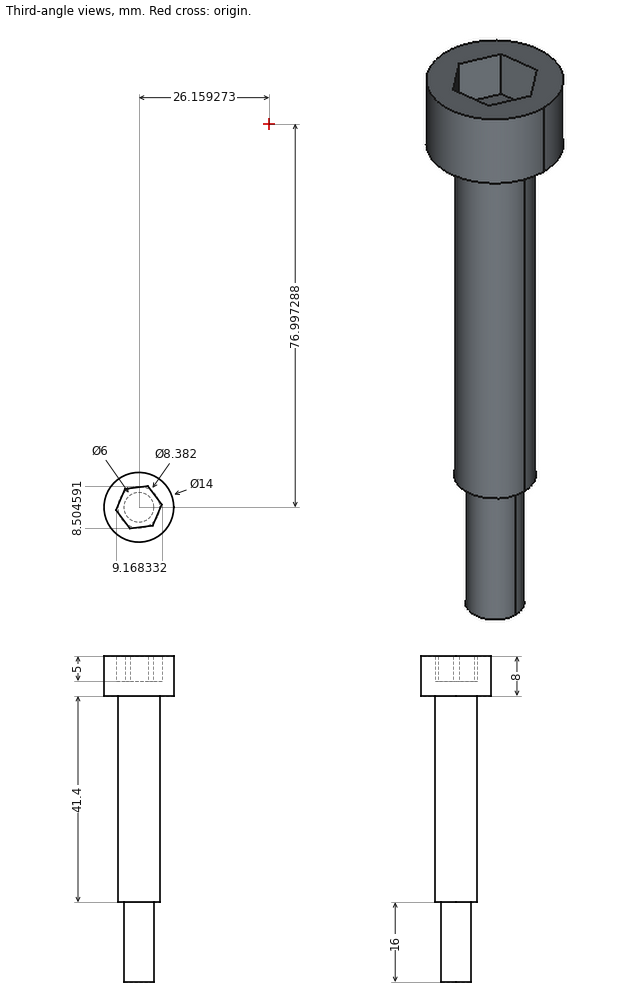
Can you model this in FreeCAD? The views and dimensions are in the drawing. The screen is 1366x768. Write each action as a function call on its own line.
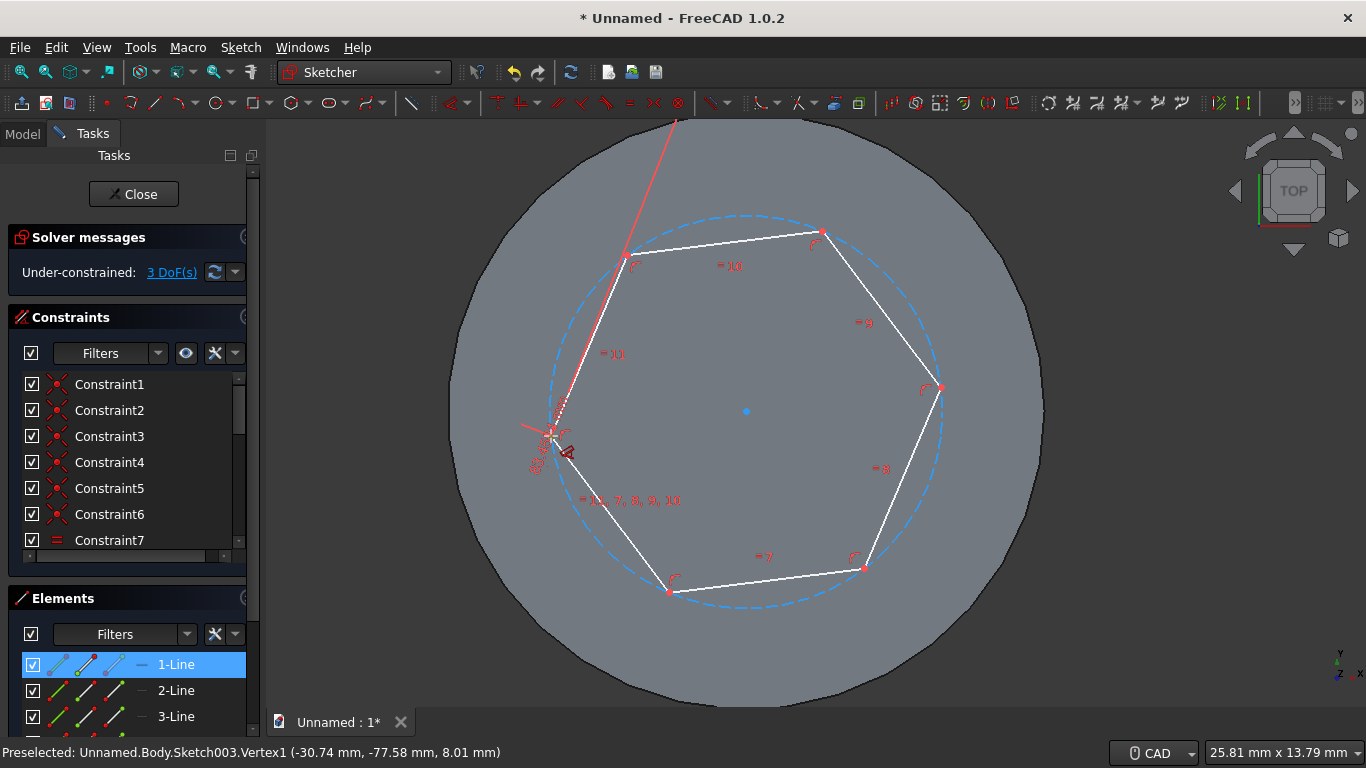
click(941, 388)
click(746, 470)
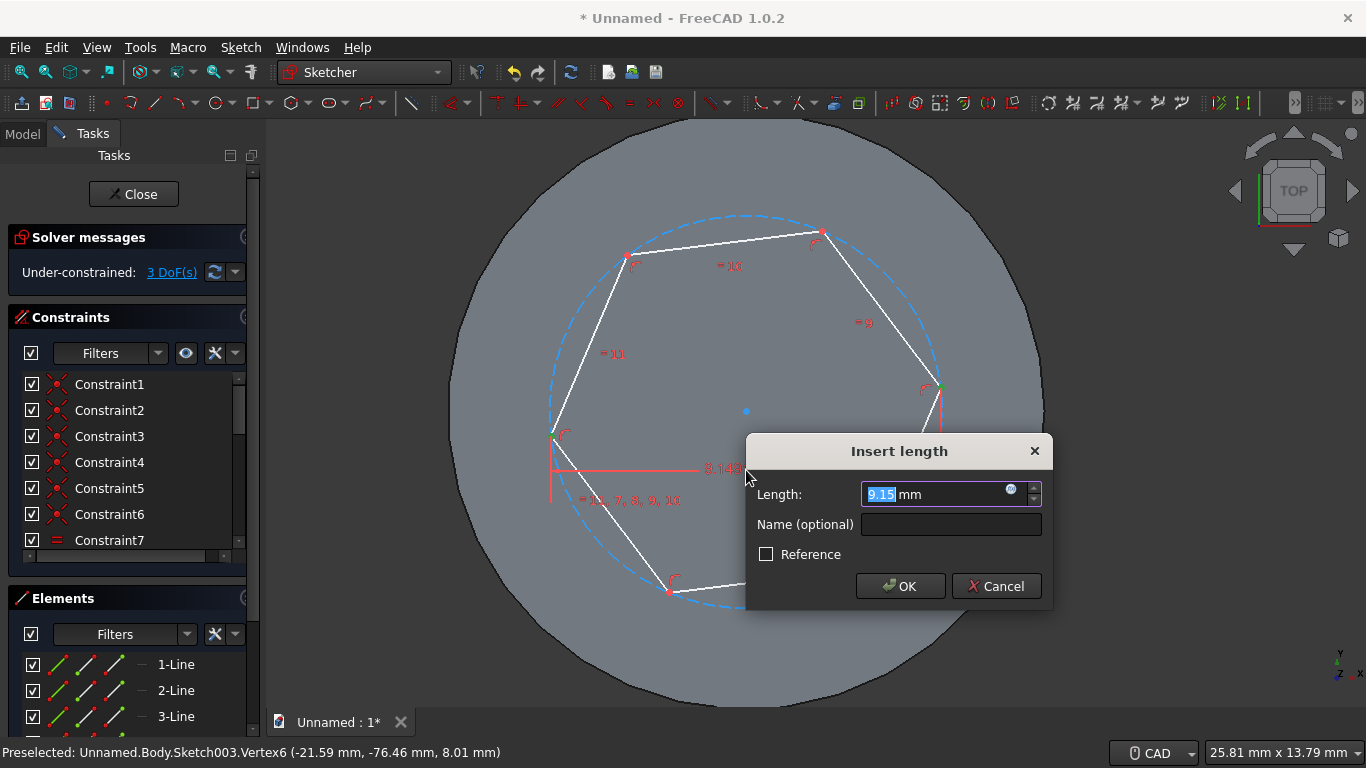
text(9.168332)
key(Return)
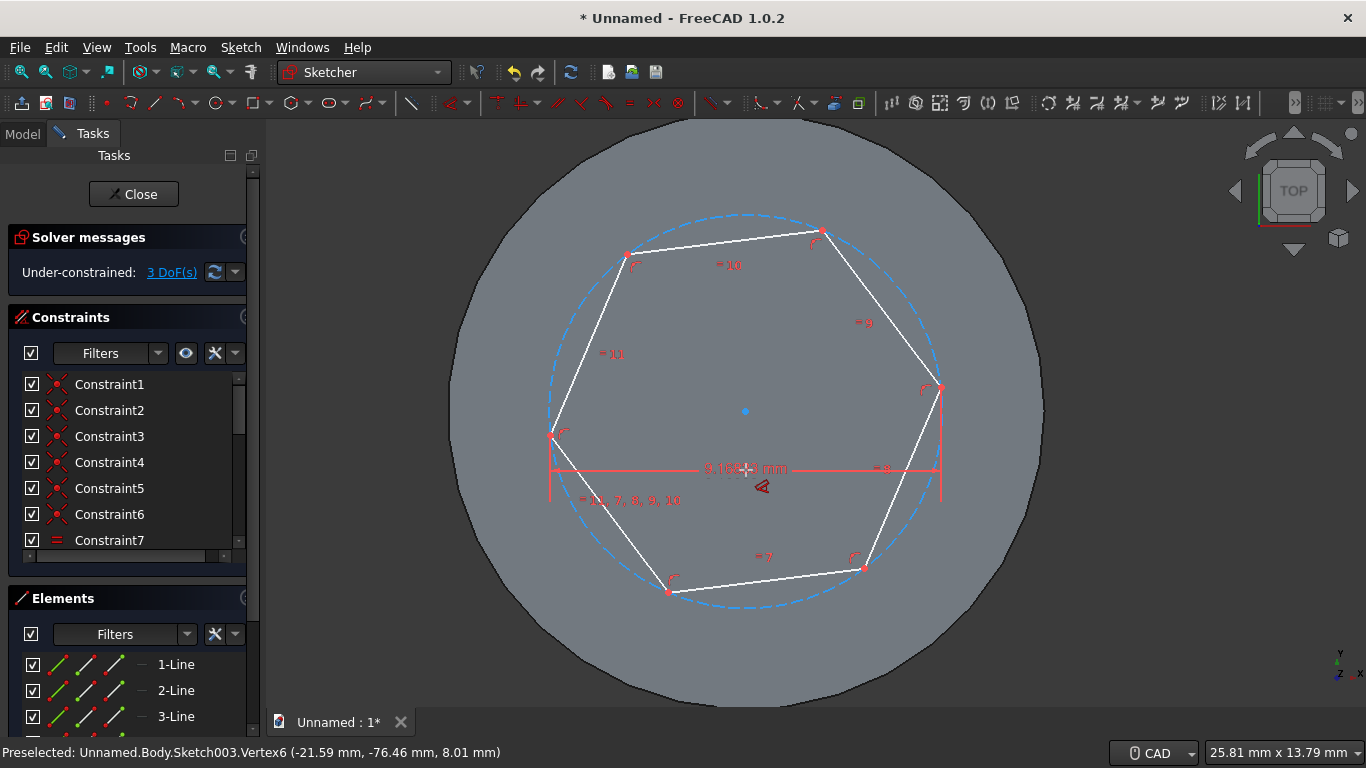
click(669, 593)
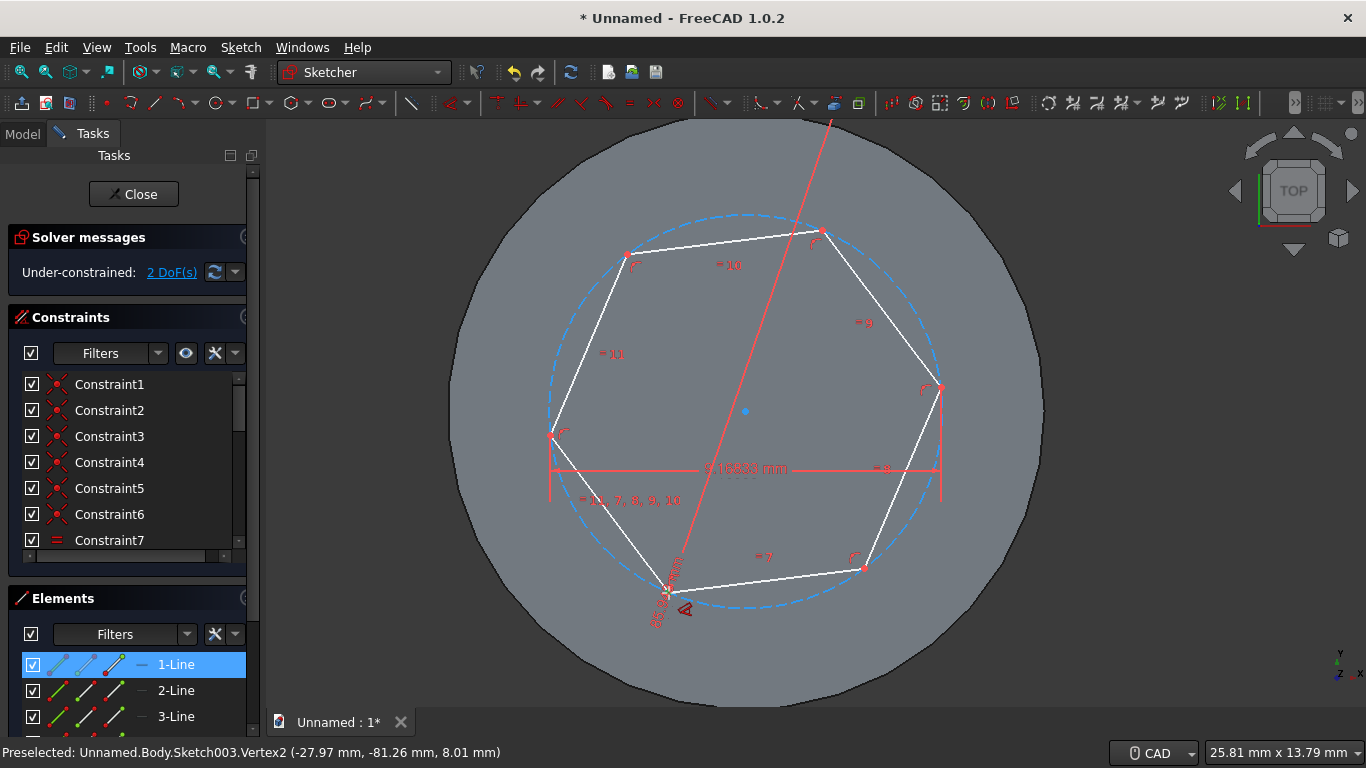
click(823, 230)
click(635, 412)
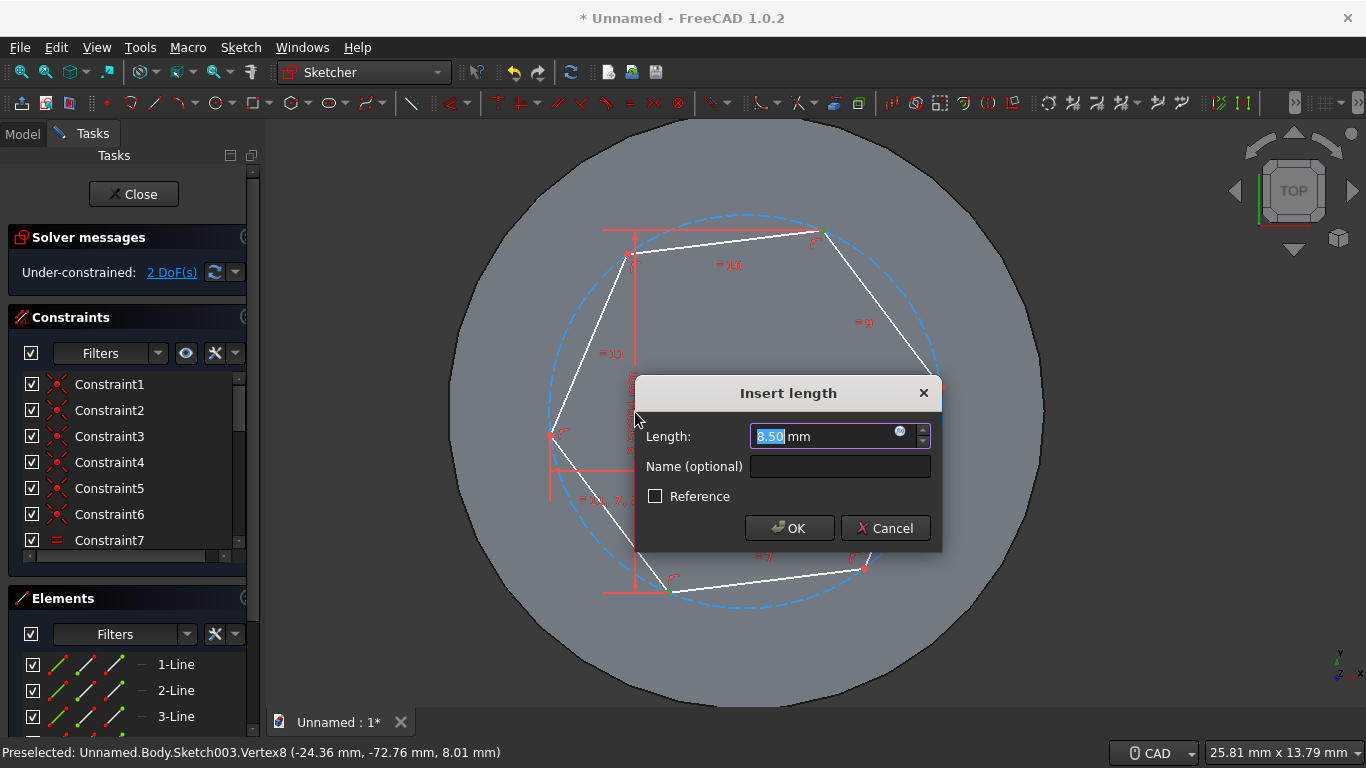
text(8.504591)
key(Return)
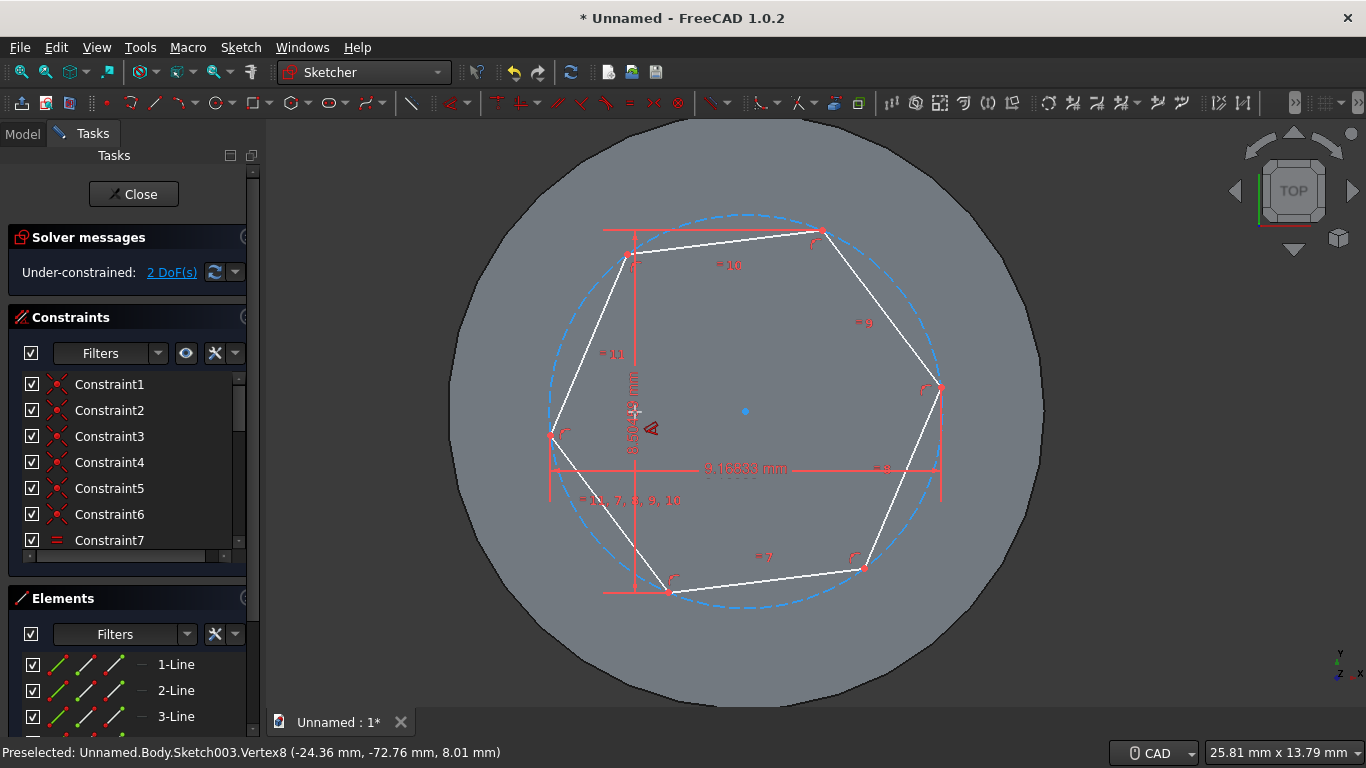
click(746, 412)
click(973, 446)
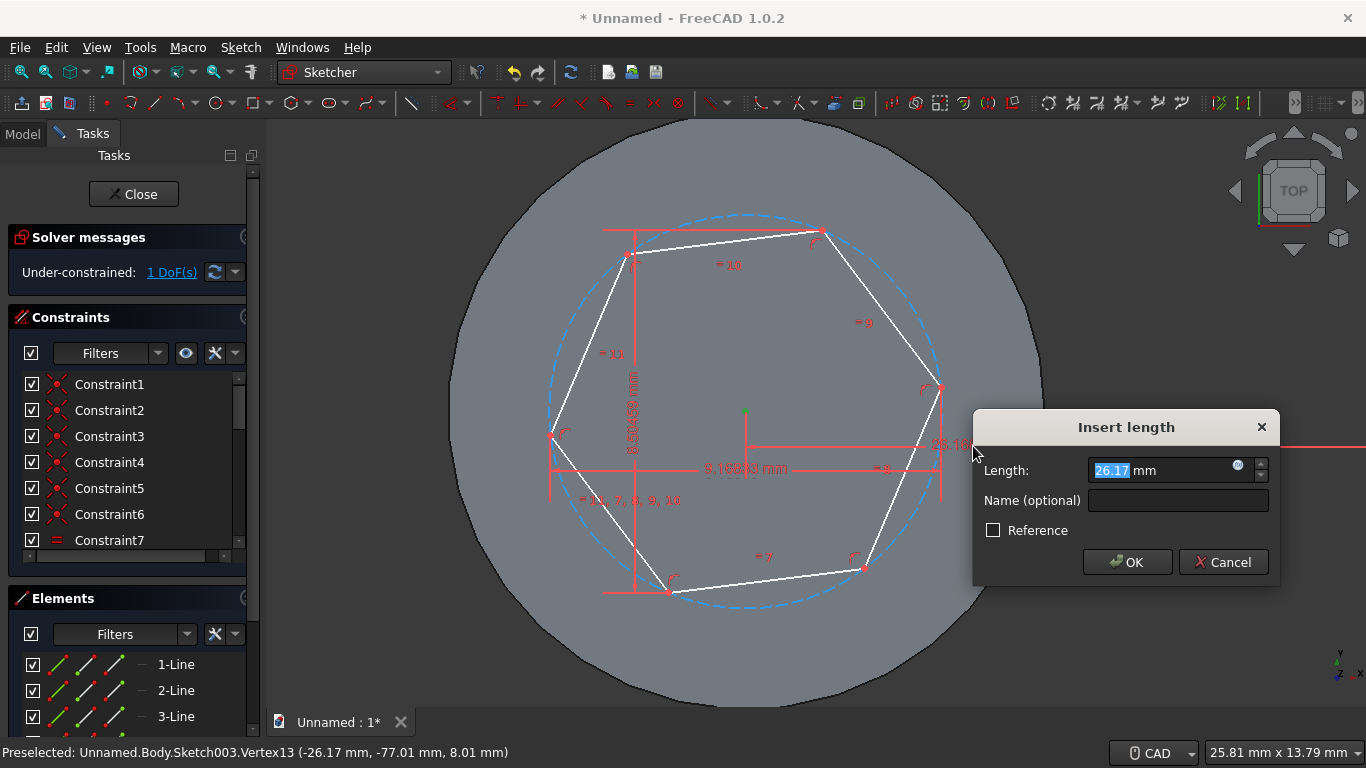
text(26.159273)
key(Return)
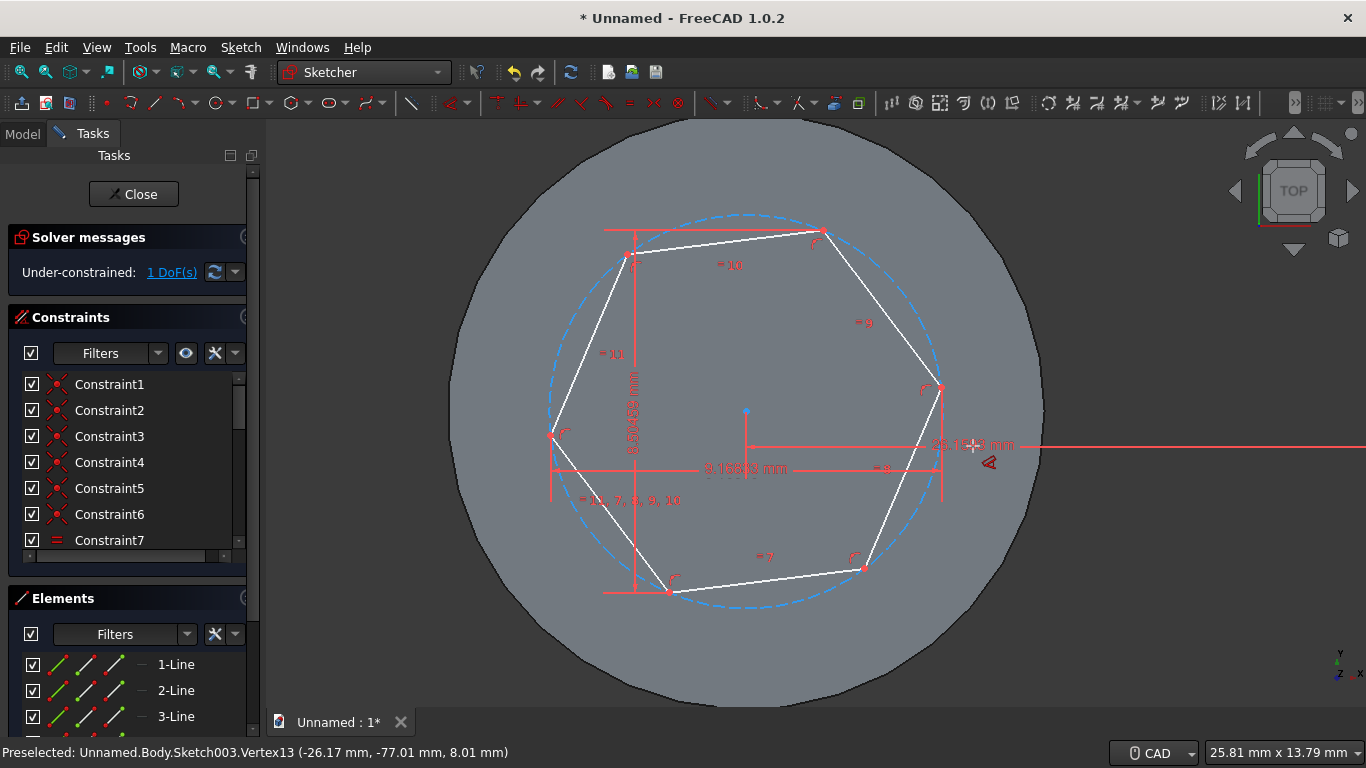
click(746, 412)
click(712, 279)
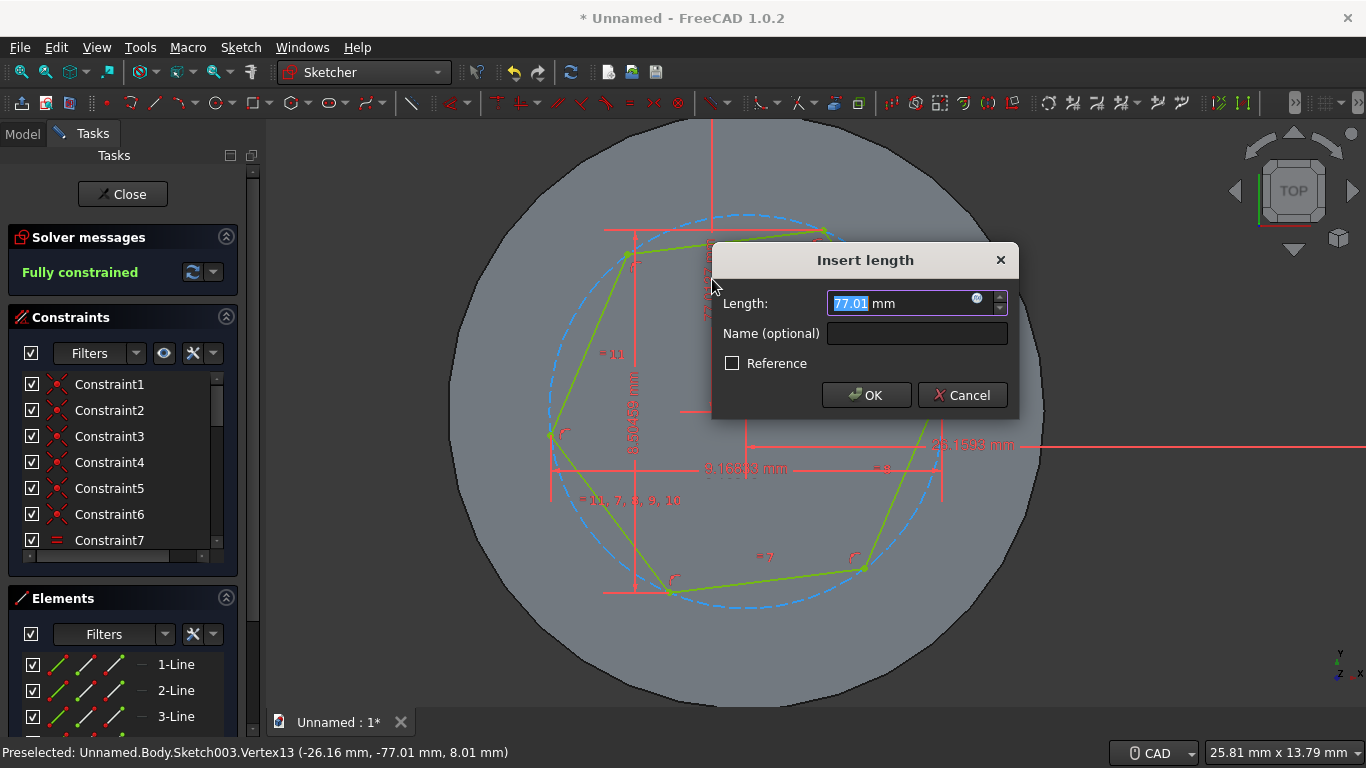
text(76.997288)
key(Return)
key(Escape)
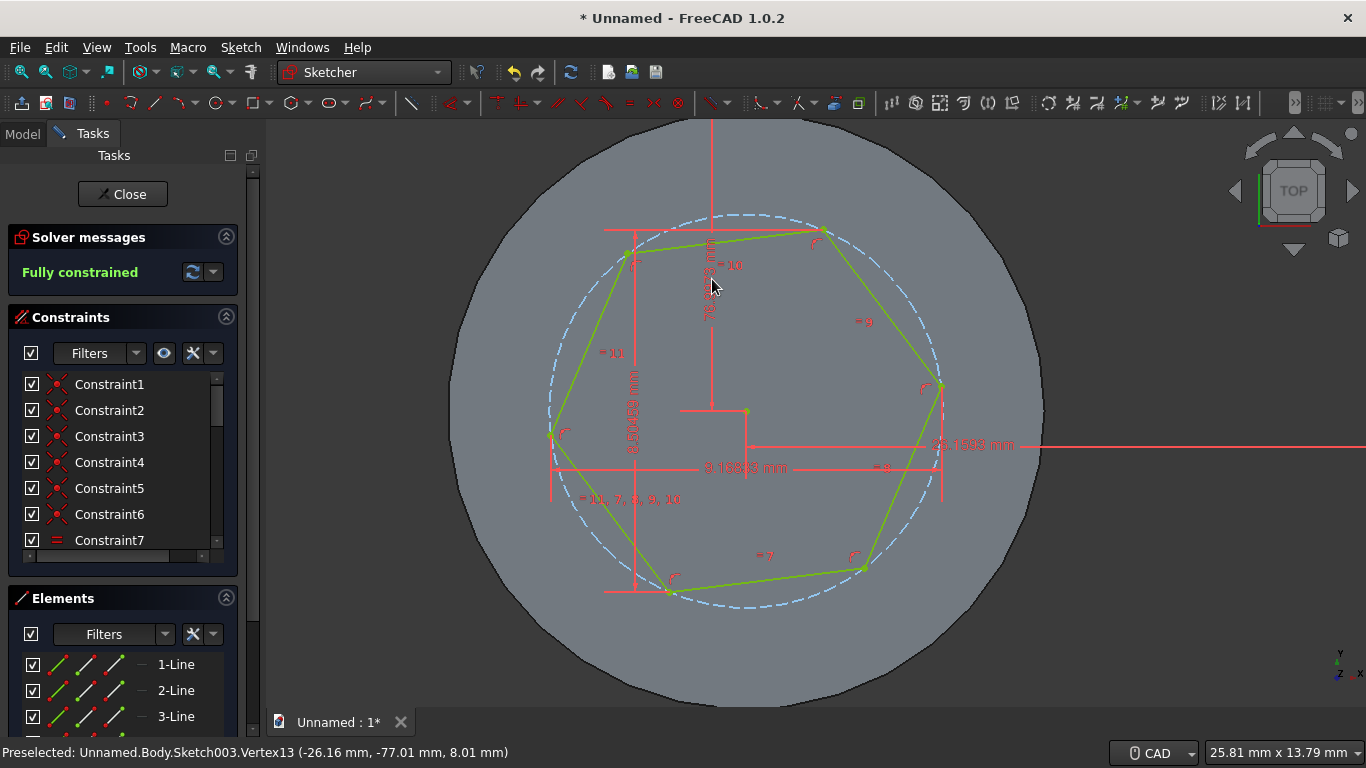
click(123, 194)